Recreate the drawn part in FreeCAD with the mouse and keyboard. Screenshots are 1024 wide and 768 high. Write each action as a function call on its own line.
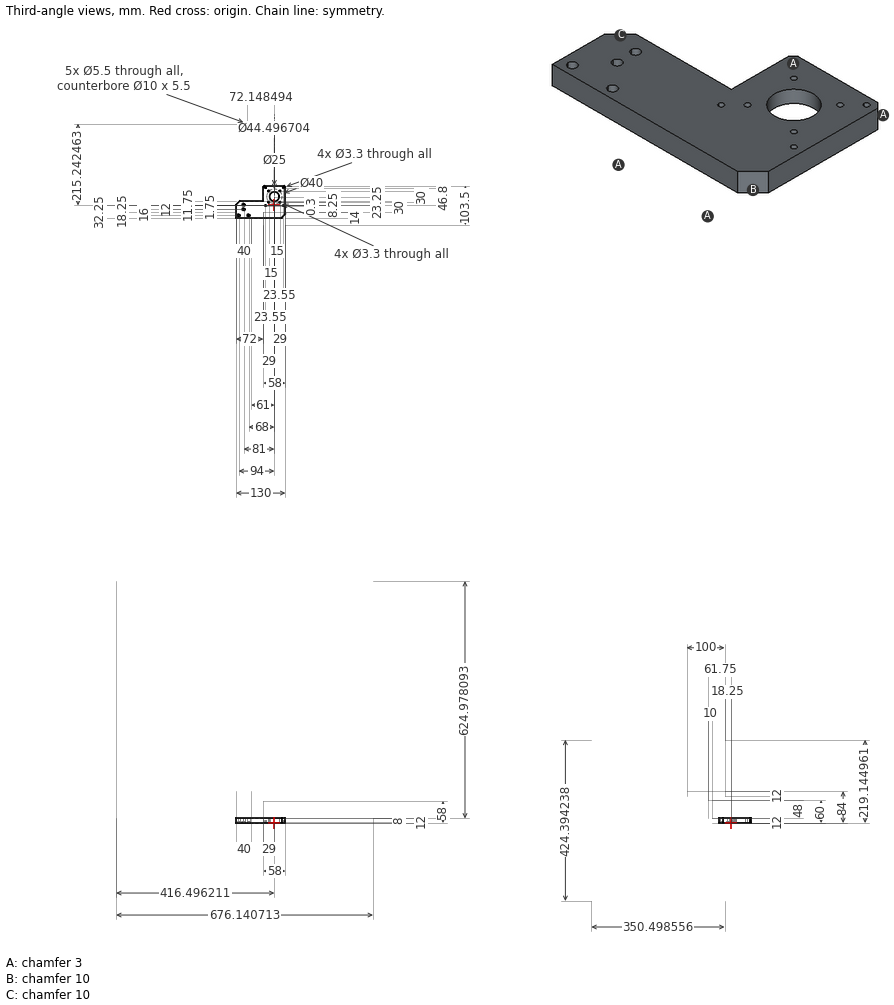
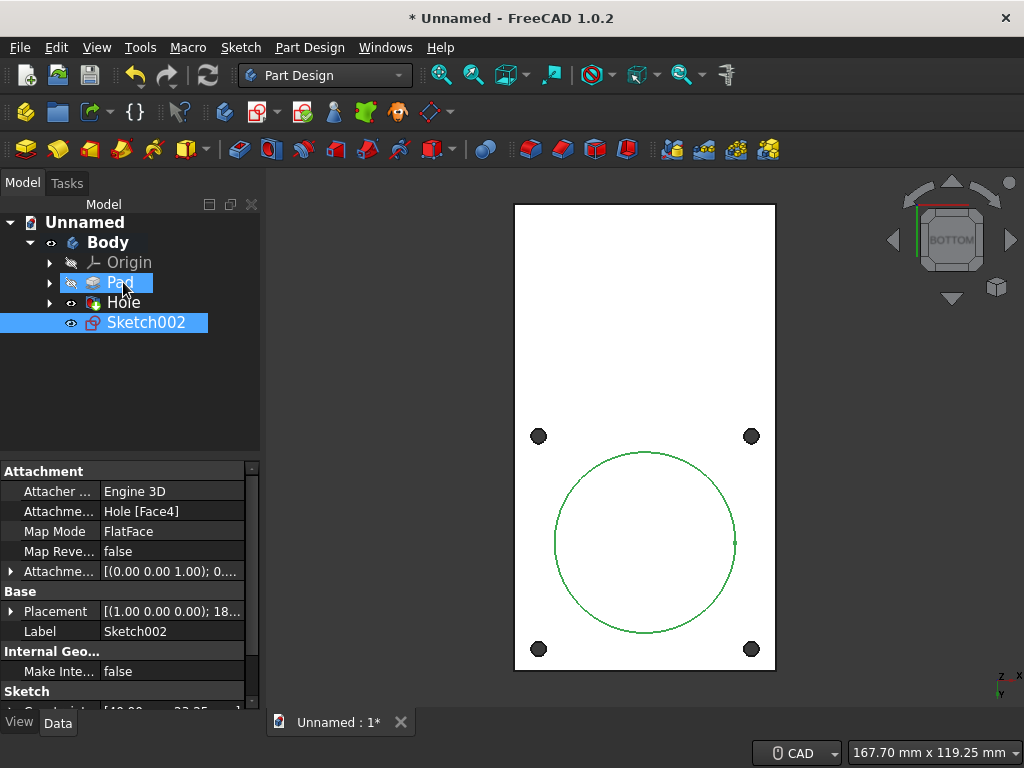
click(240, 150)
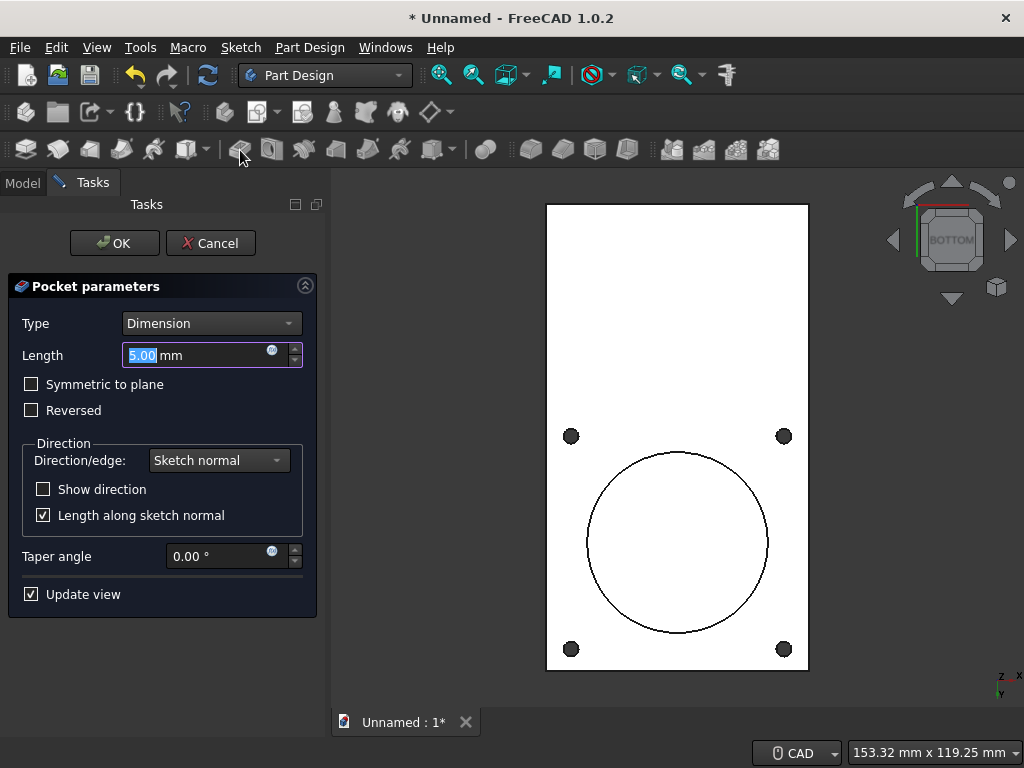
click(212, 324)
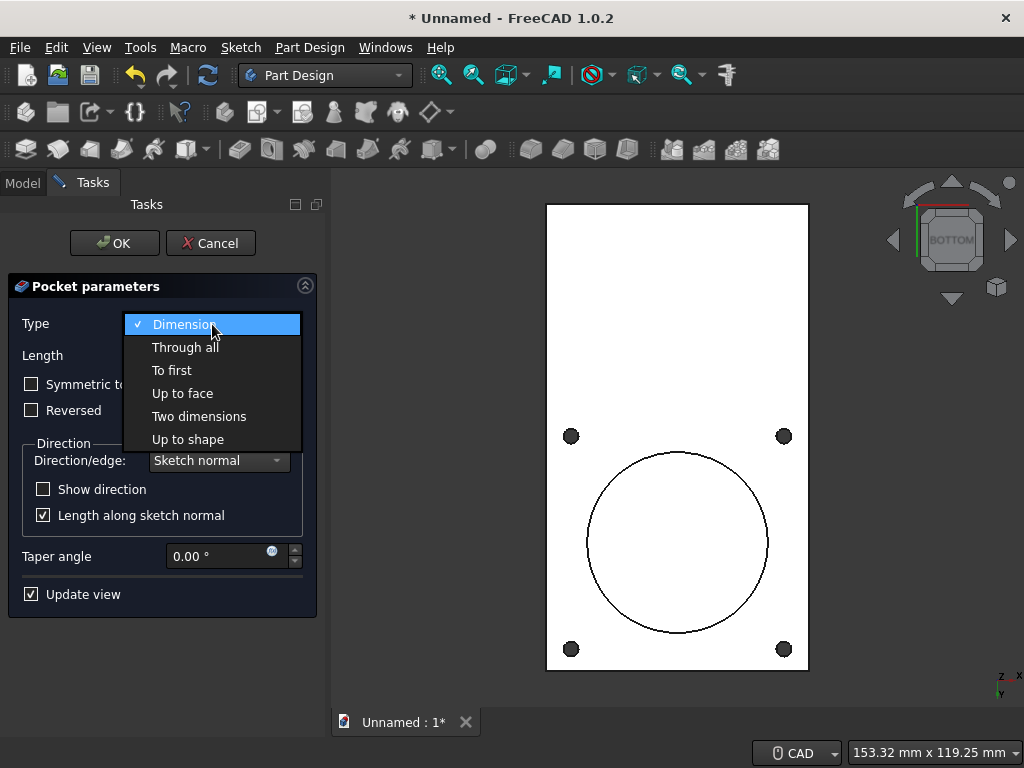
click(212, 348)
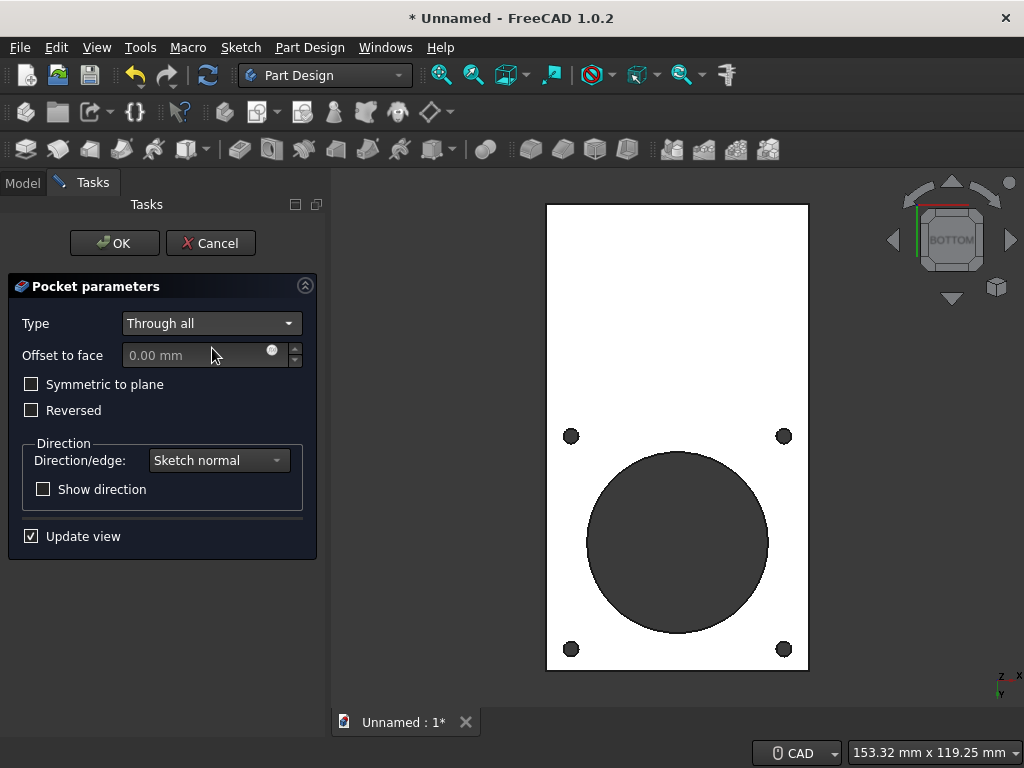
click(115, 243)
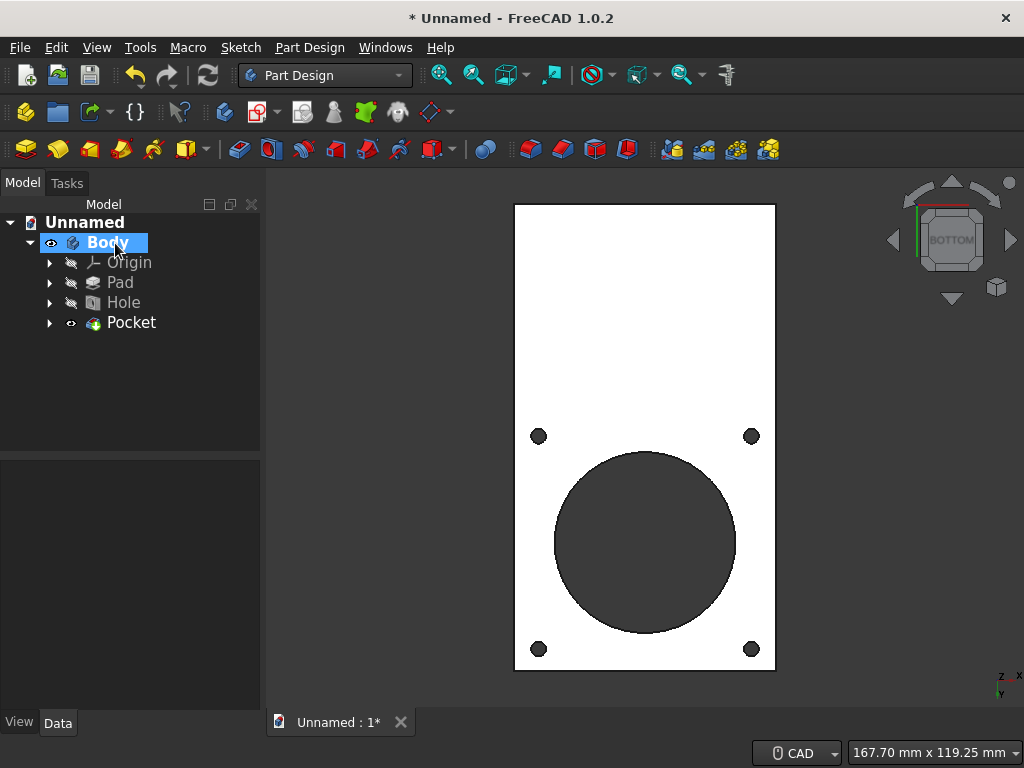
key(0)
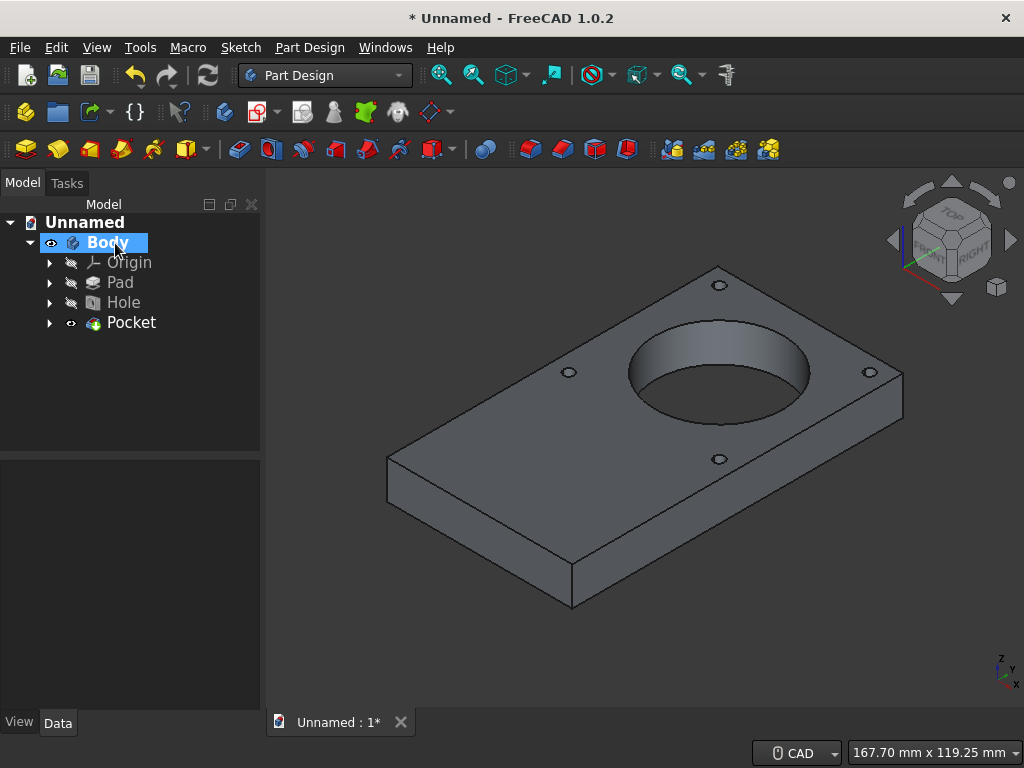
click(533, 563)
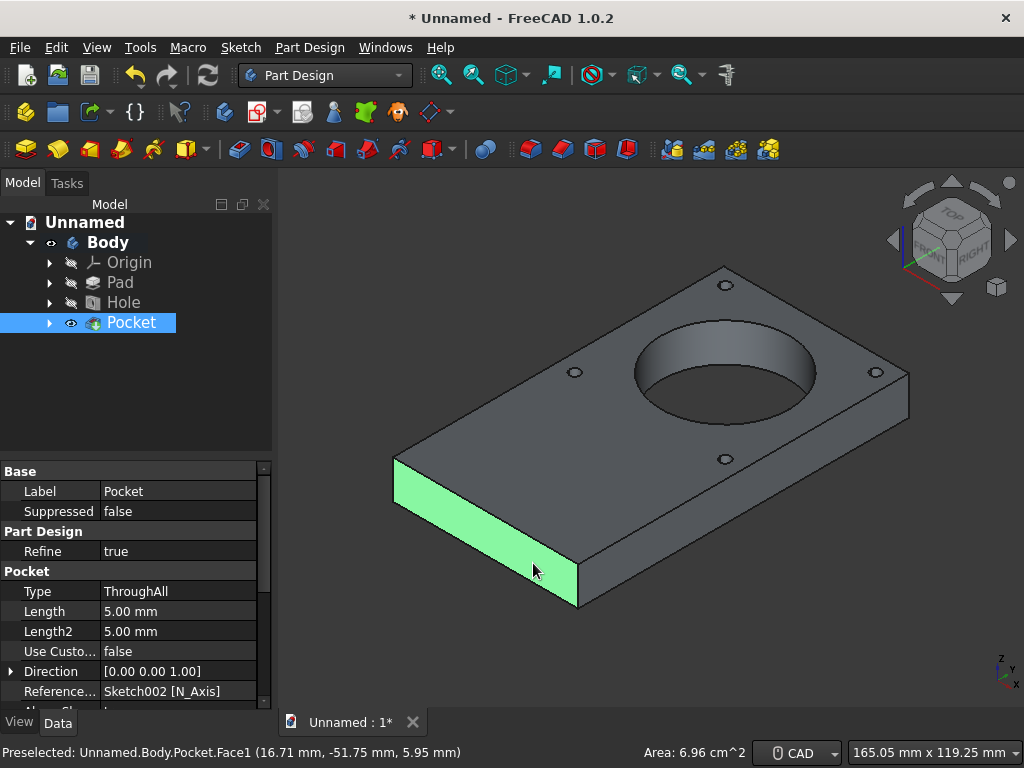
click(258, 112)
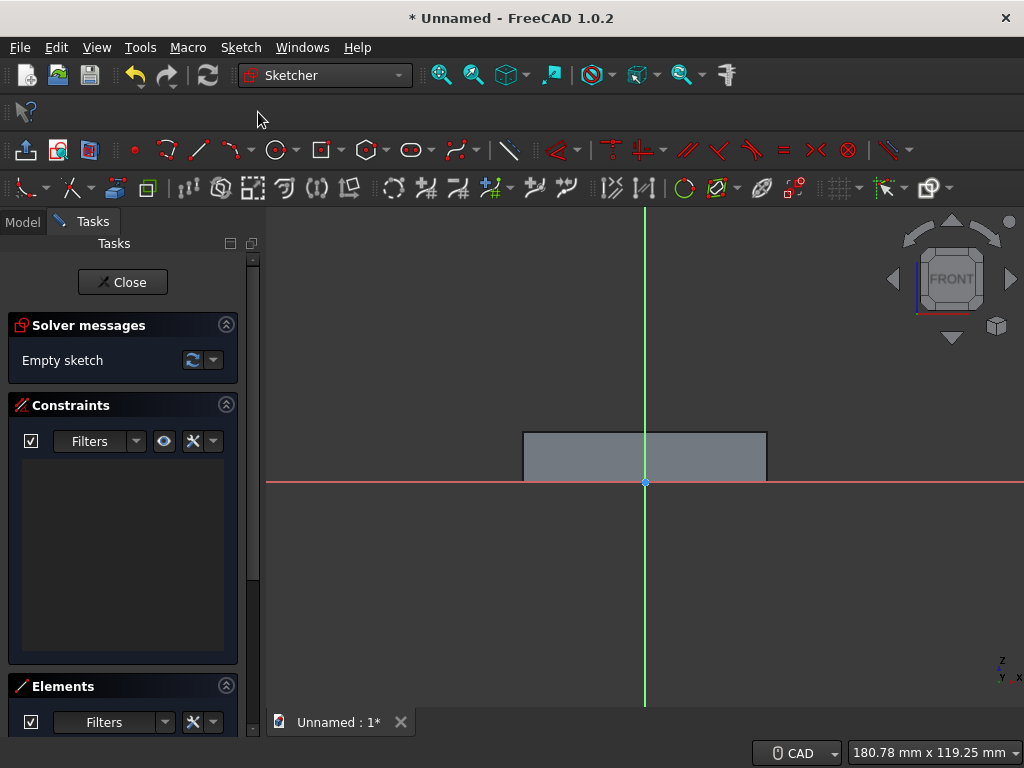
scroll(294, 679, down, 1)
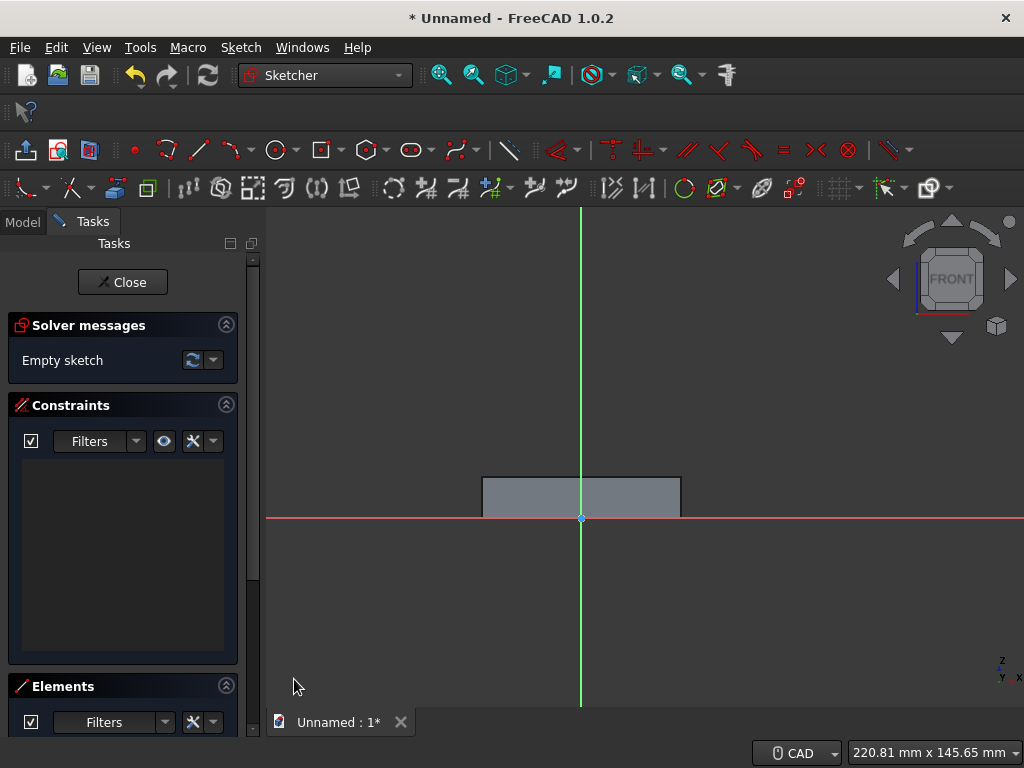
scroll(591, 340, up, 2)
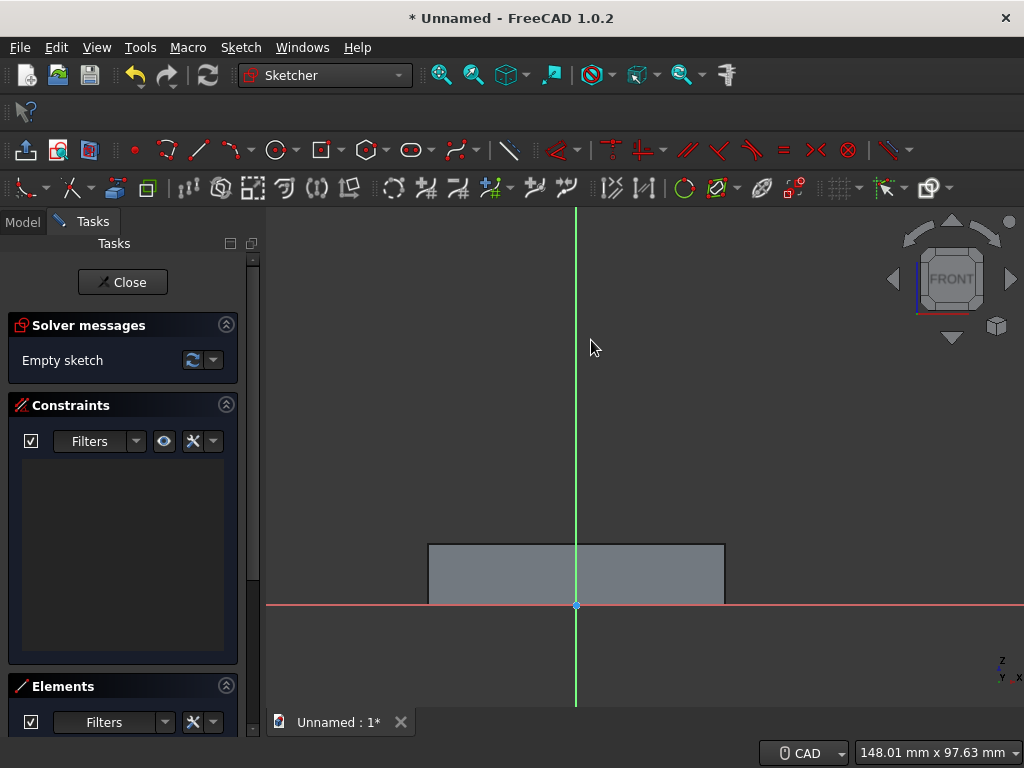
key(g)
key(r)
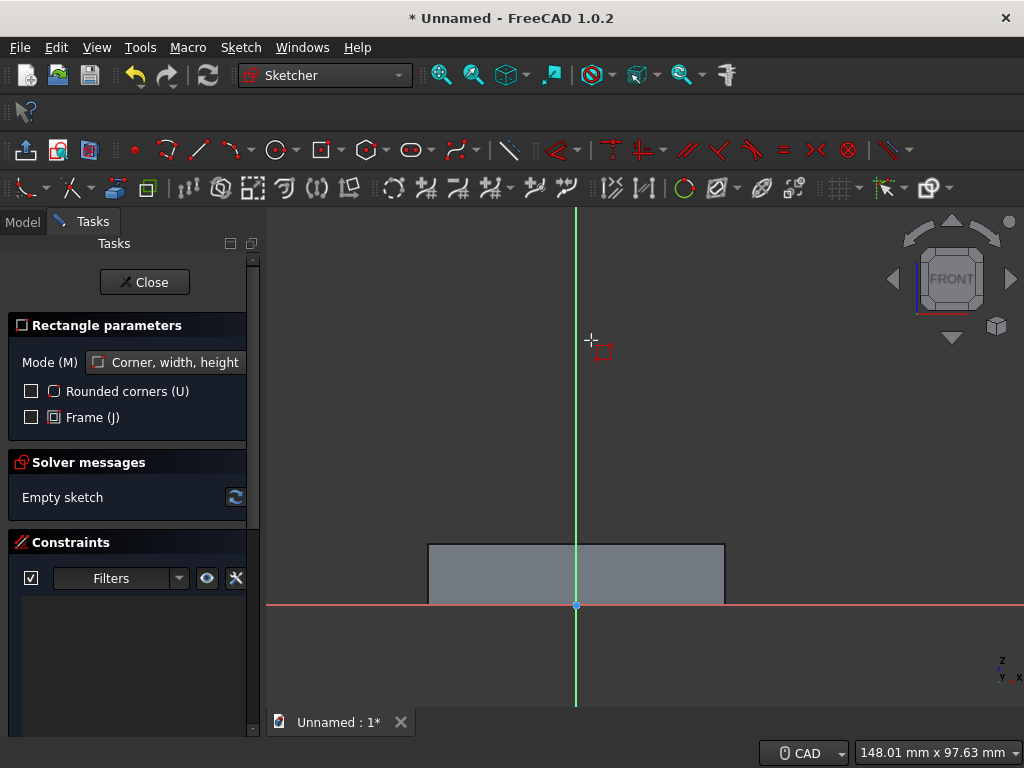
click(428, 308)
click(725, 605)
key(Escape)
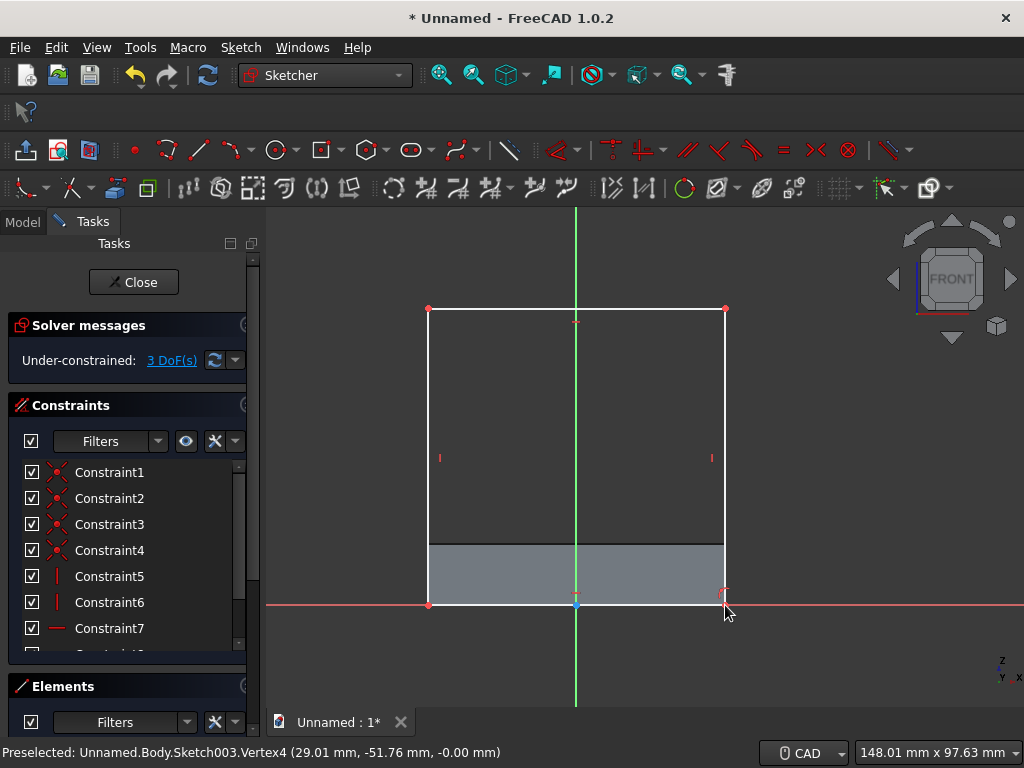
click(556, 150)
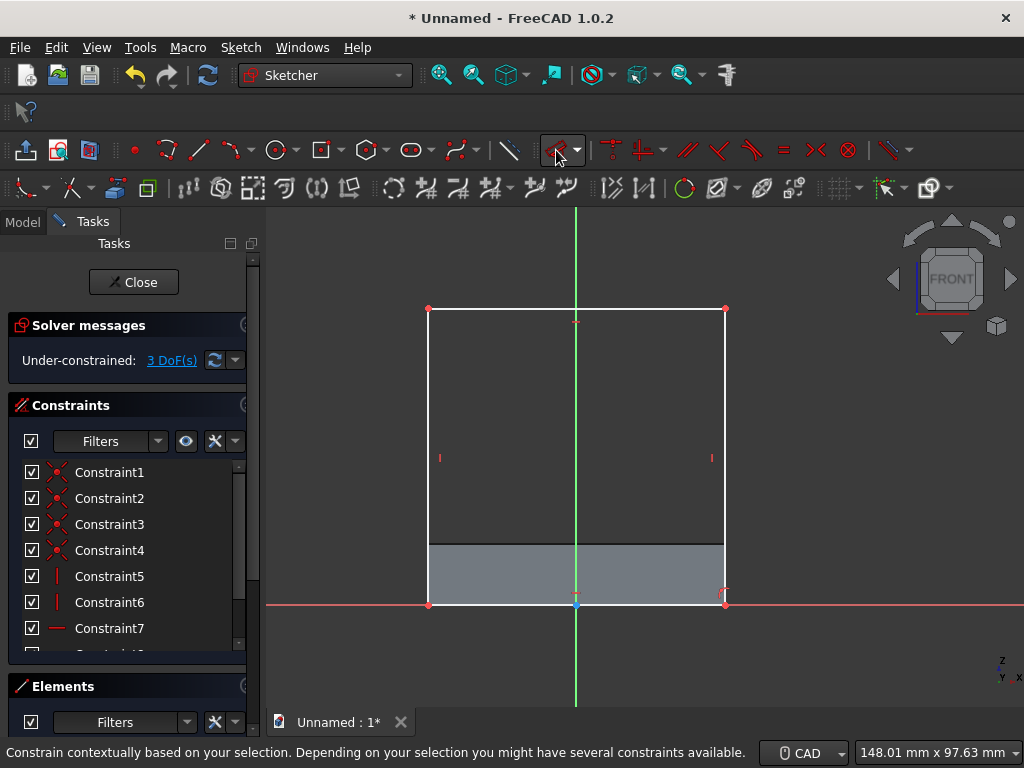
click(428, 398)
click(394, 457)